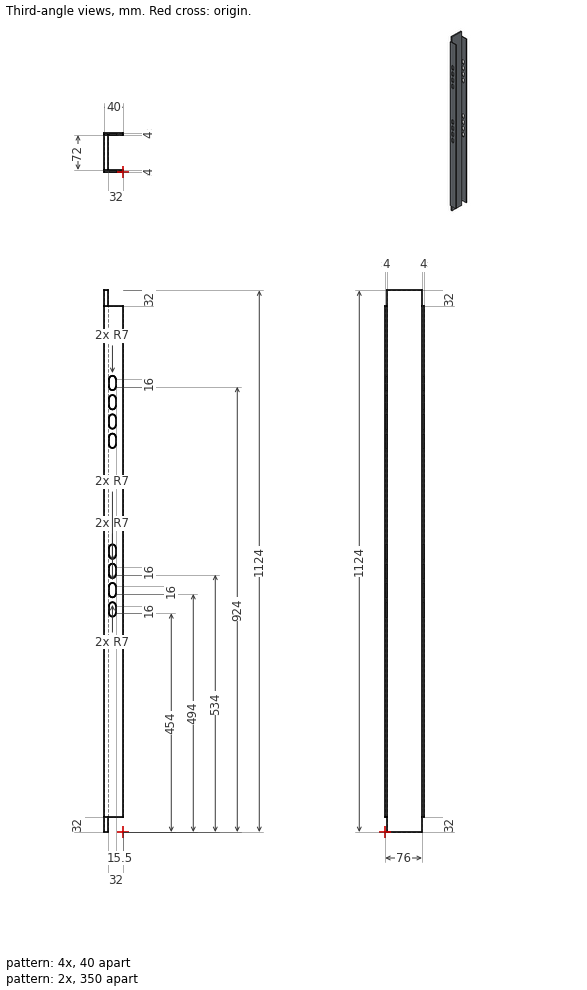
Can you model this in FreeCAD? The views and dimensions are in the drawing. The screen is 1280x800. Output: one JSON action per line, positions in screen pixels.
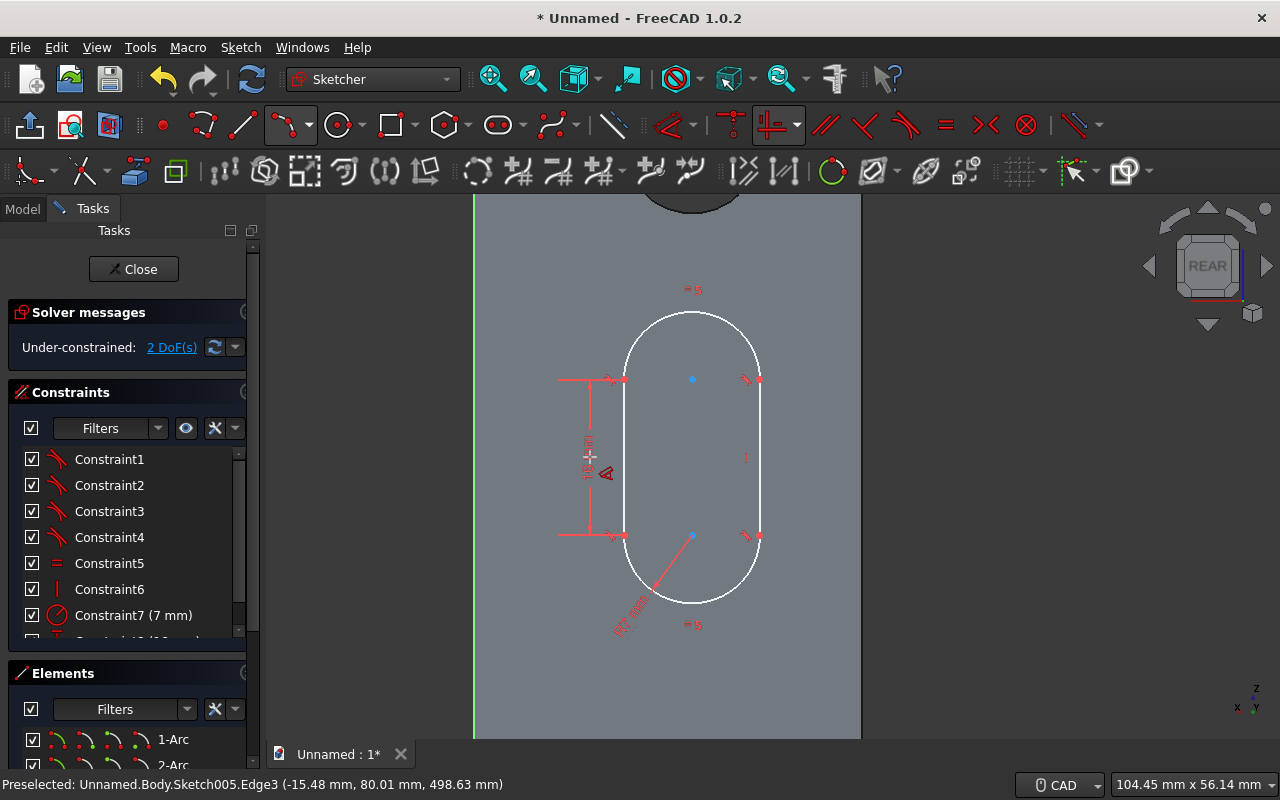
{"action": "left_click", "coordinate": [624, 535]}
{"action": "left_click", "coordinate": [440, 623]}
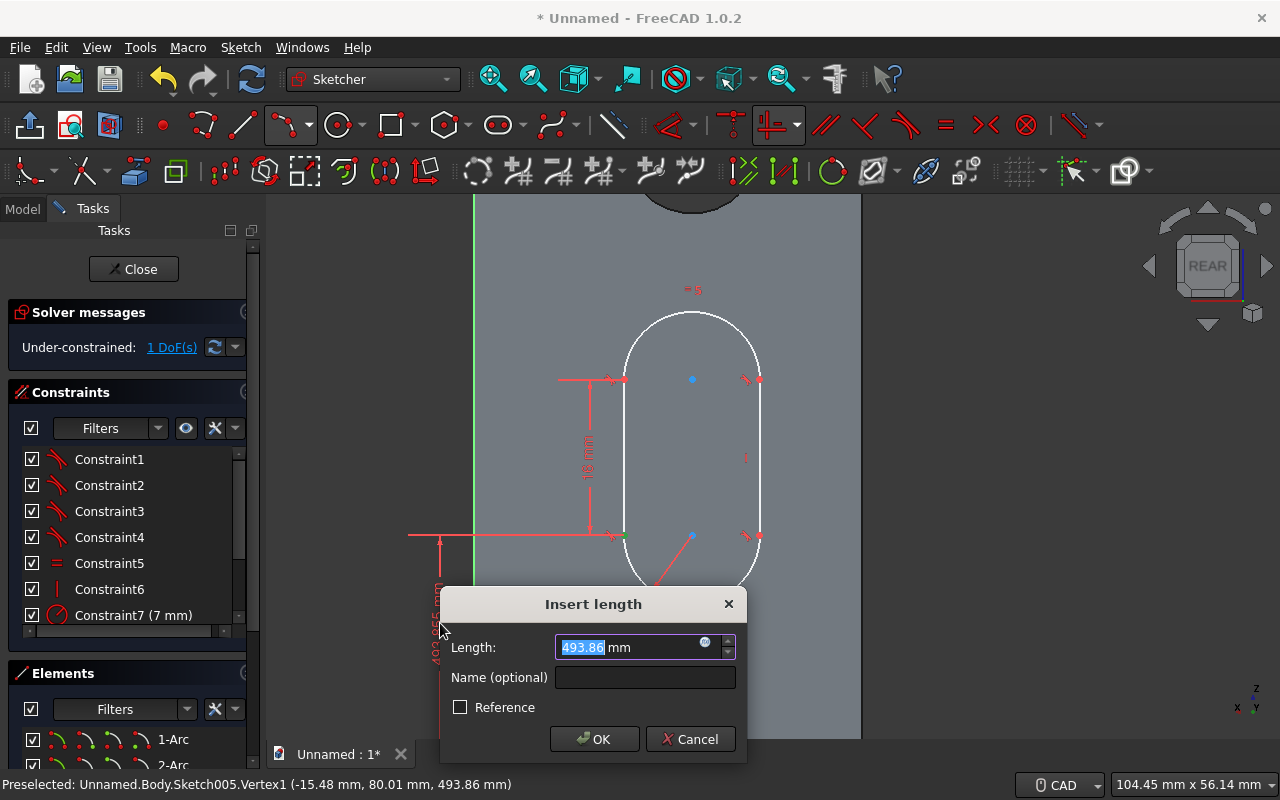
{"action": "type", "text": "494"}
{"action": "key", "text": "Return"}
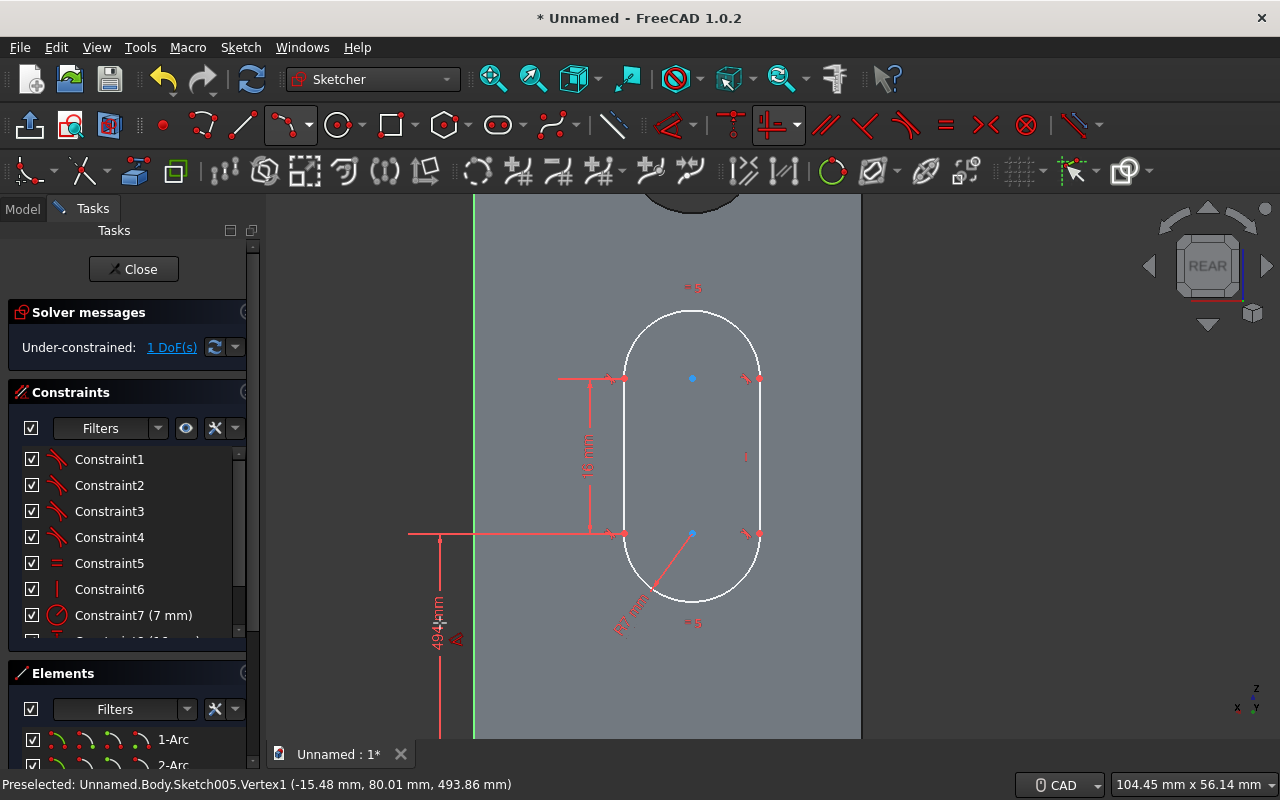
{"action": "left_click", "coordinate": [624, 534]}
{"action": "left_click", "coordinate": [549, 500]}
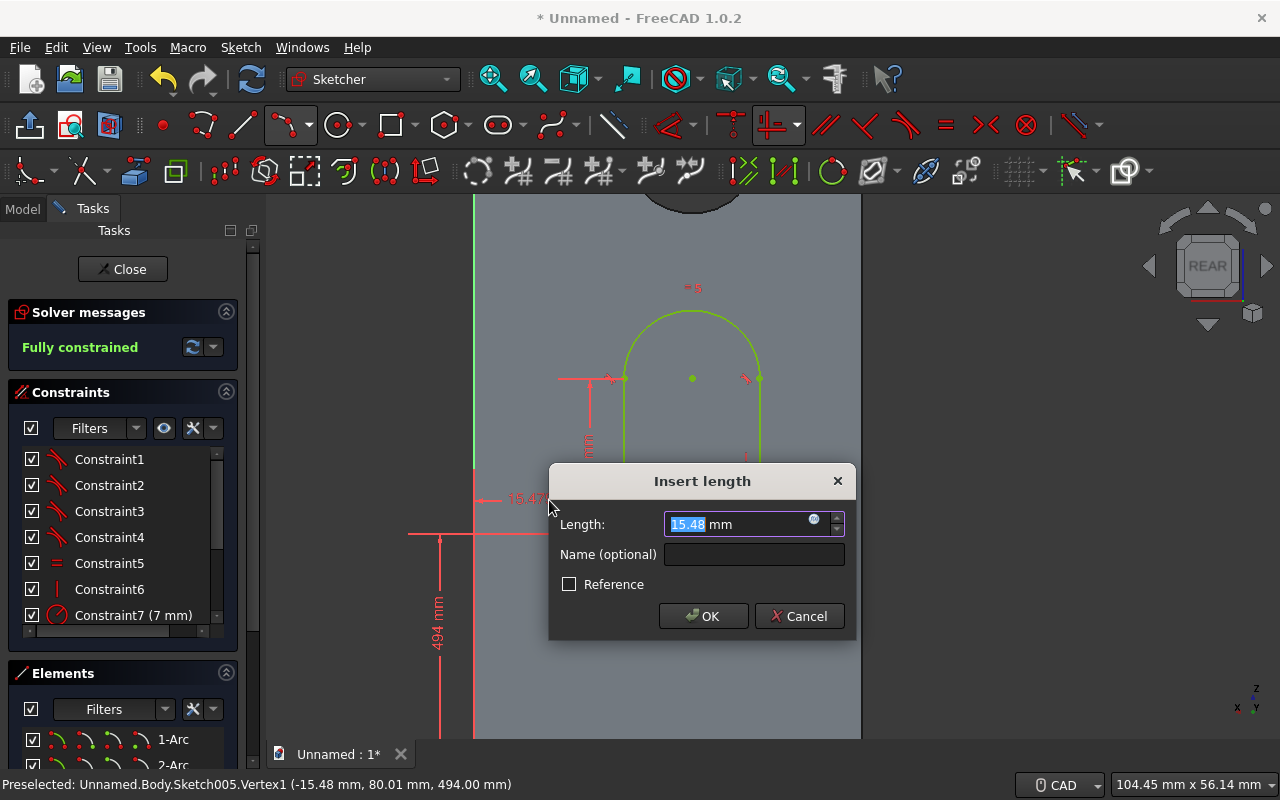
{"action": "type", "text": "15.5"}
{"action": "key", "text": "Return"}
{"action": "key", "text": "Escape"}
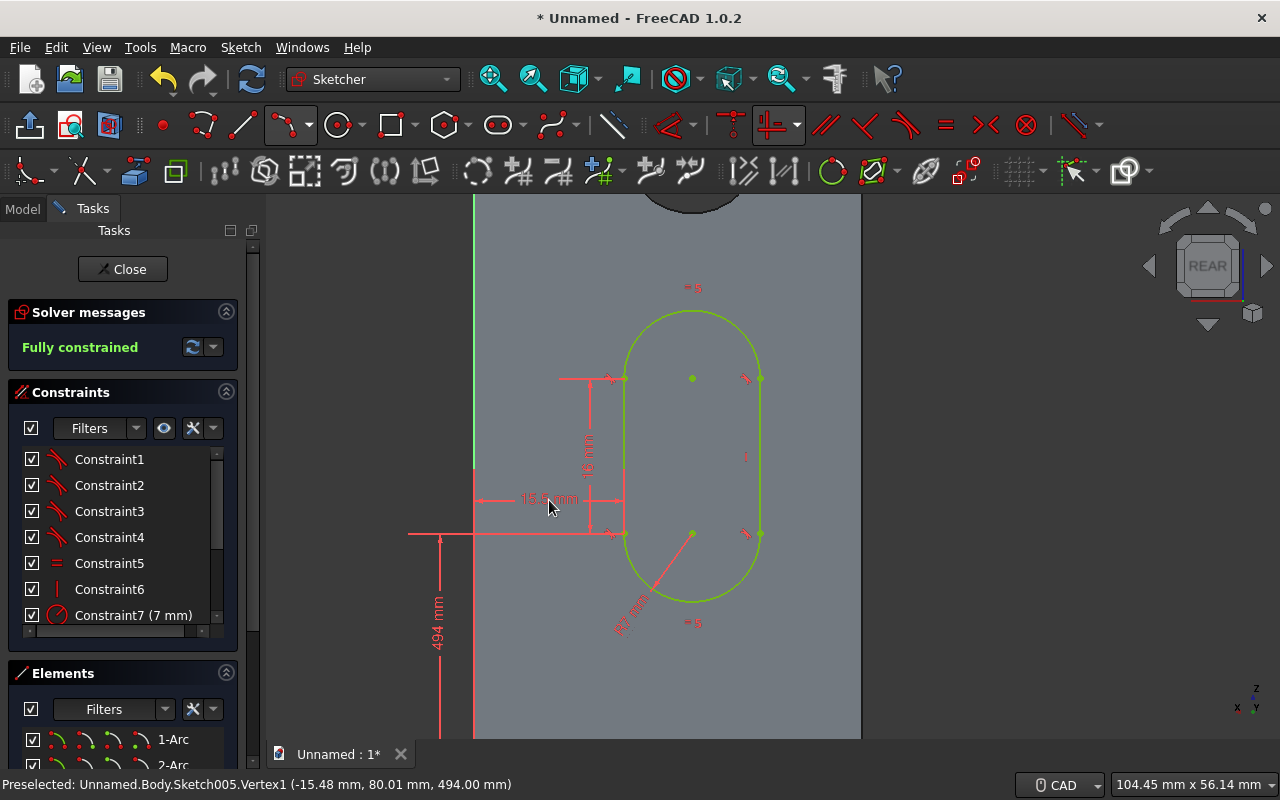
{"action": "left_click", "coordinate": [123, 269]}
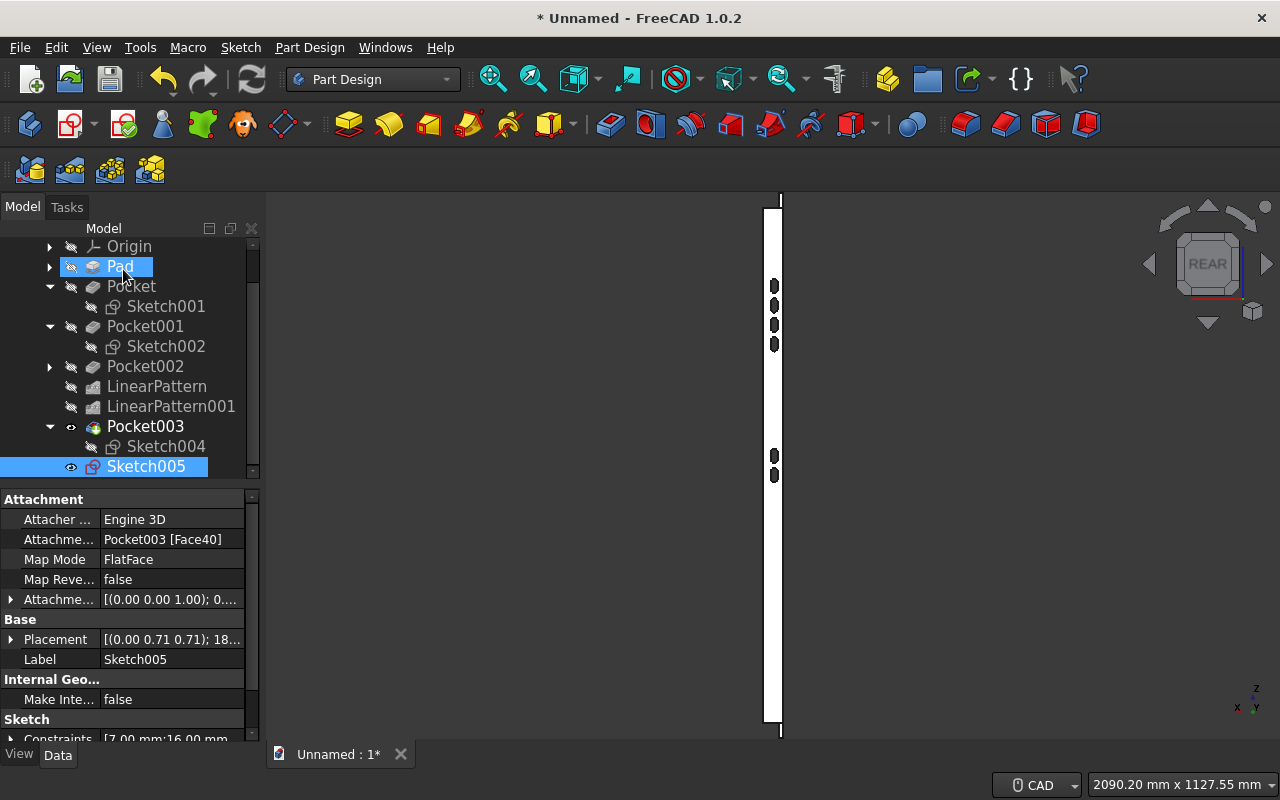
{"action": "left_click", "coordinate": [612, 124]}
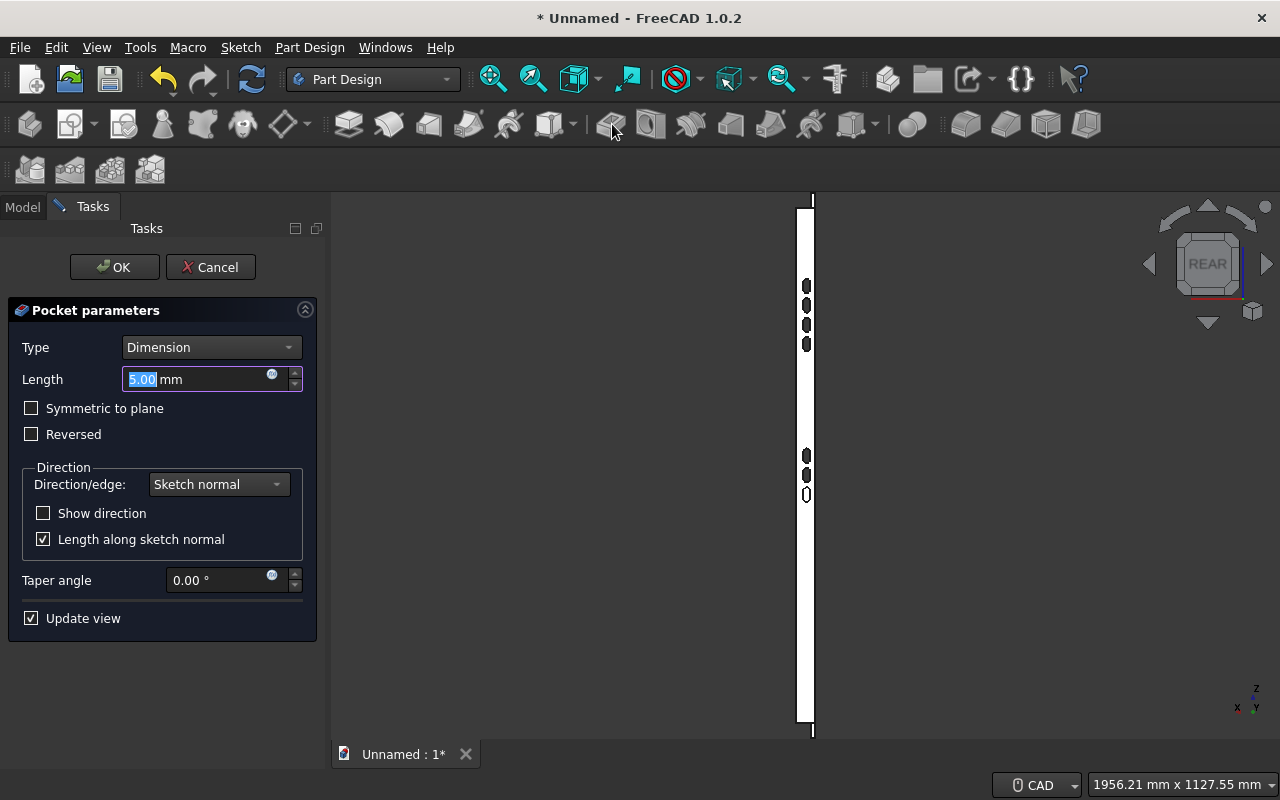
{"action": "left_click", "coordinate": [212, 348]}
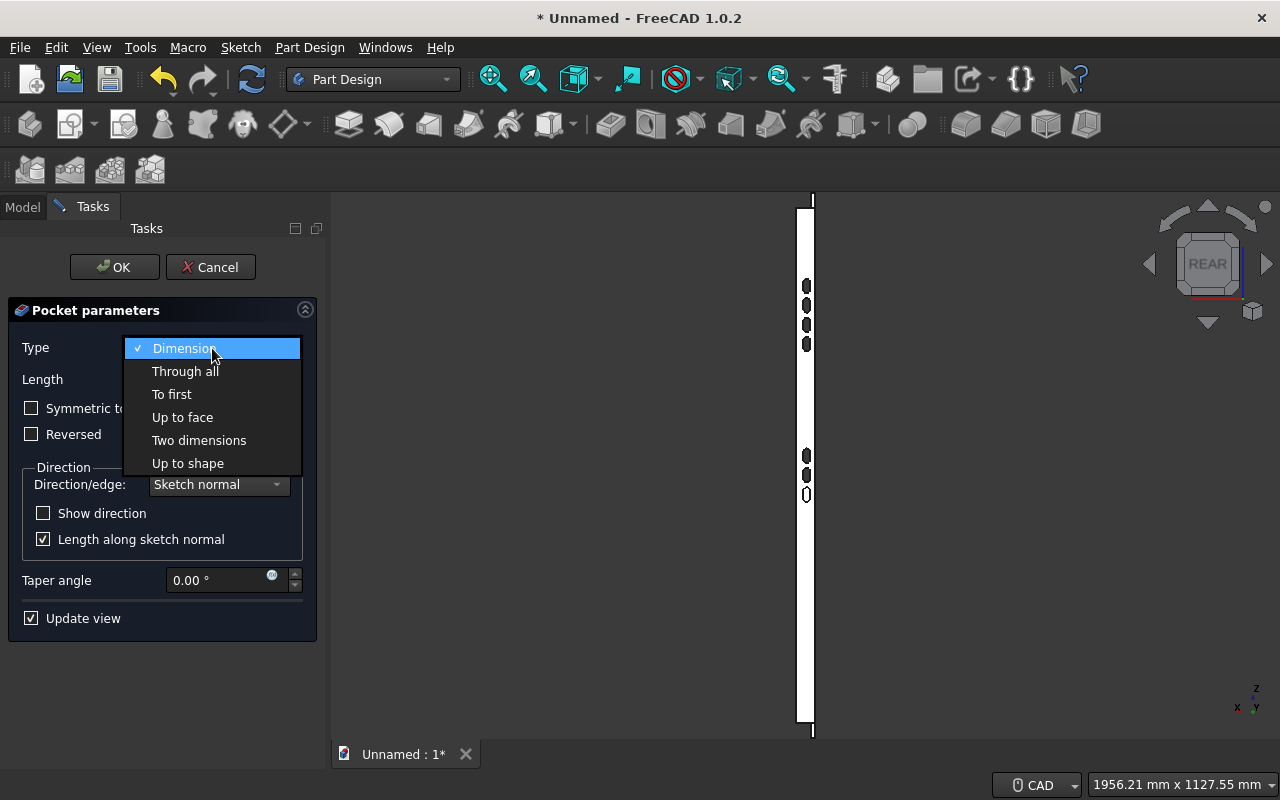
{"action": "left_click", "coordinate": [212, 372]}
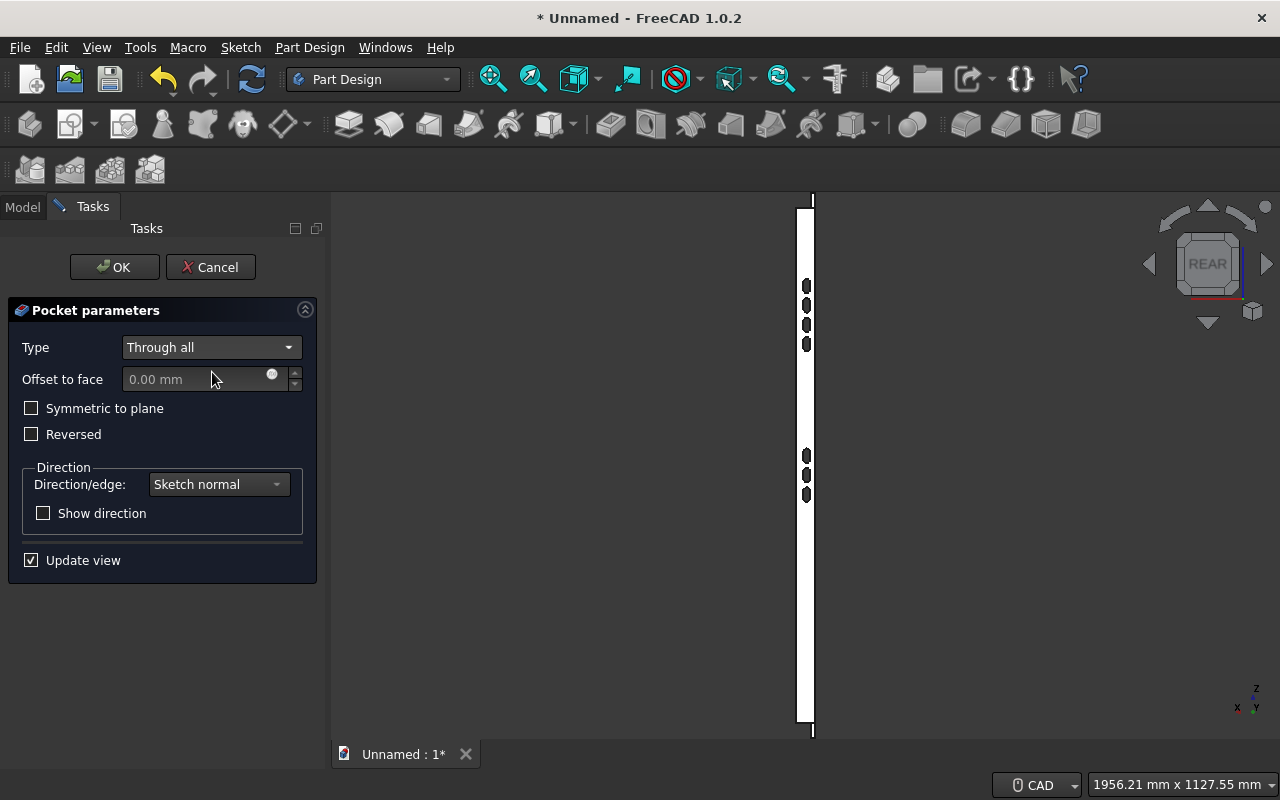
{"action": "left_click", "coordinate": [115, 267]}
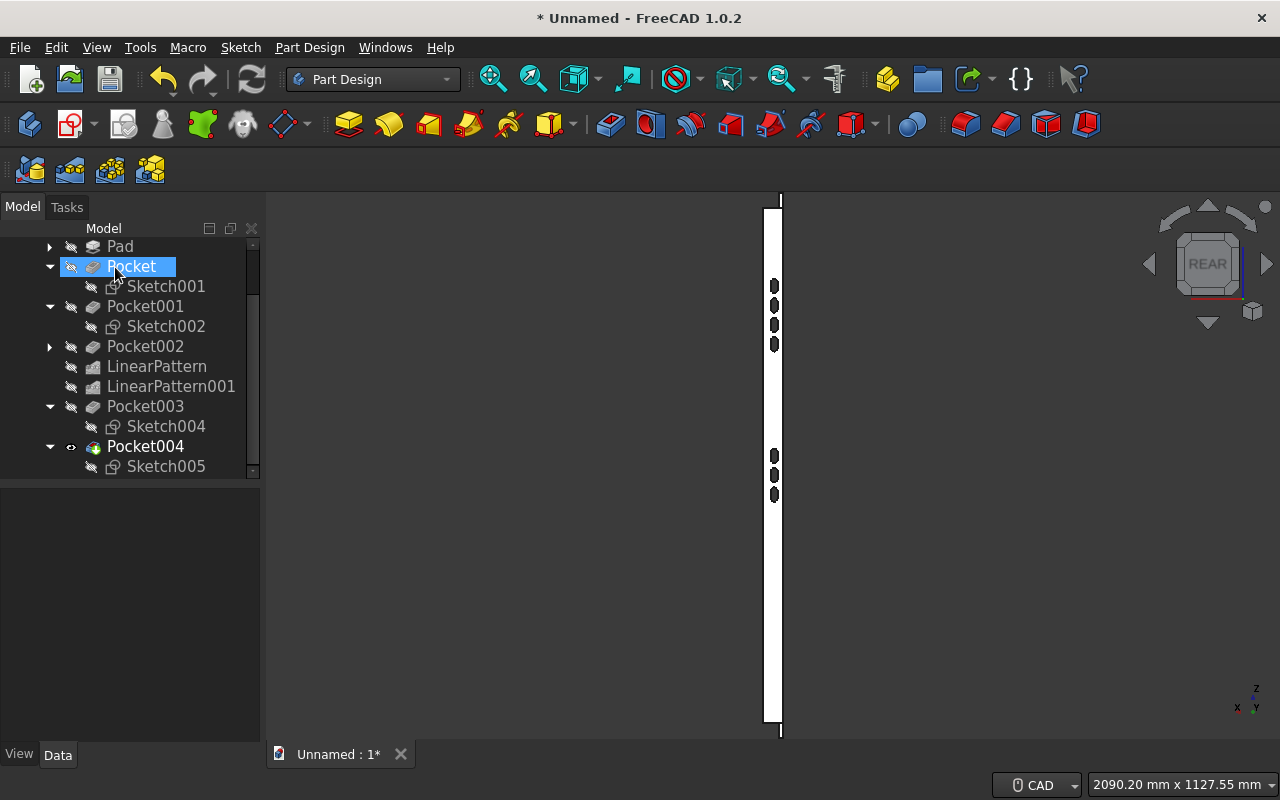
{"action": "left_click", "coordinate": [773, 244]}